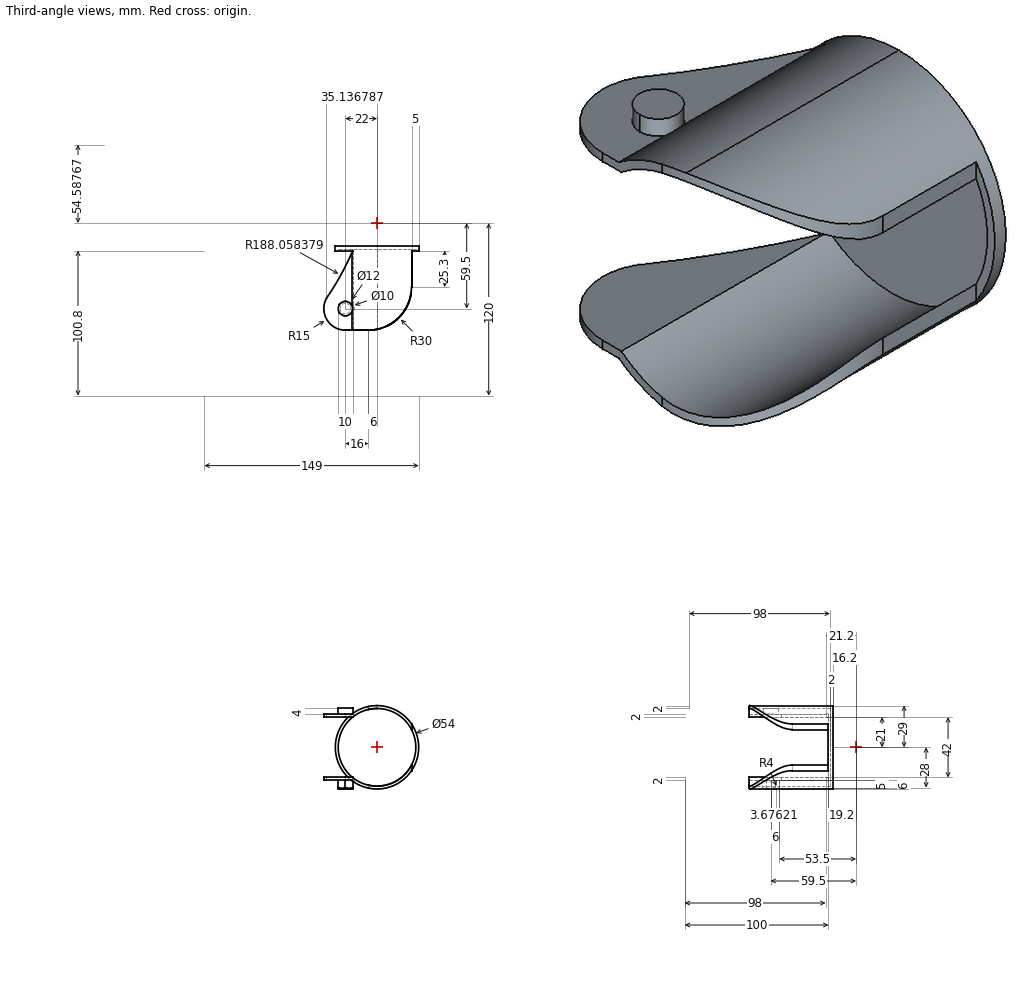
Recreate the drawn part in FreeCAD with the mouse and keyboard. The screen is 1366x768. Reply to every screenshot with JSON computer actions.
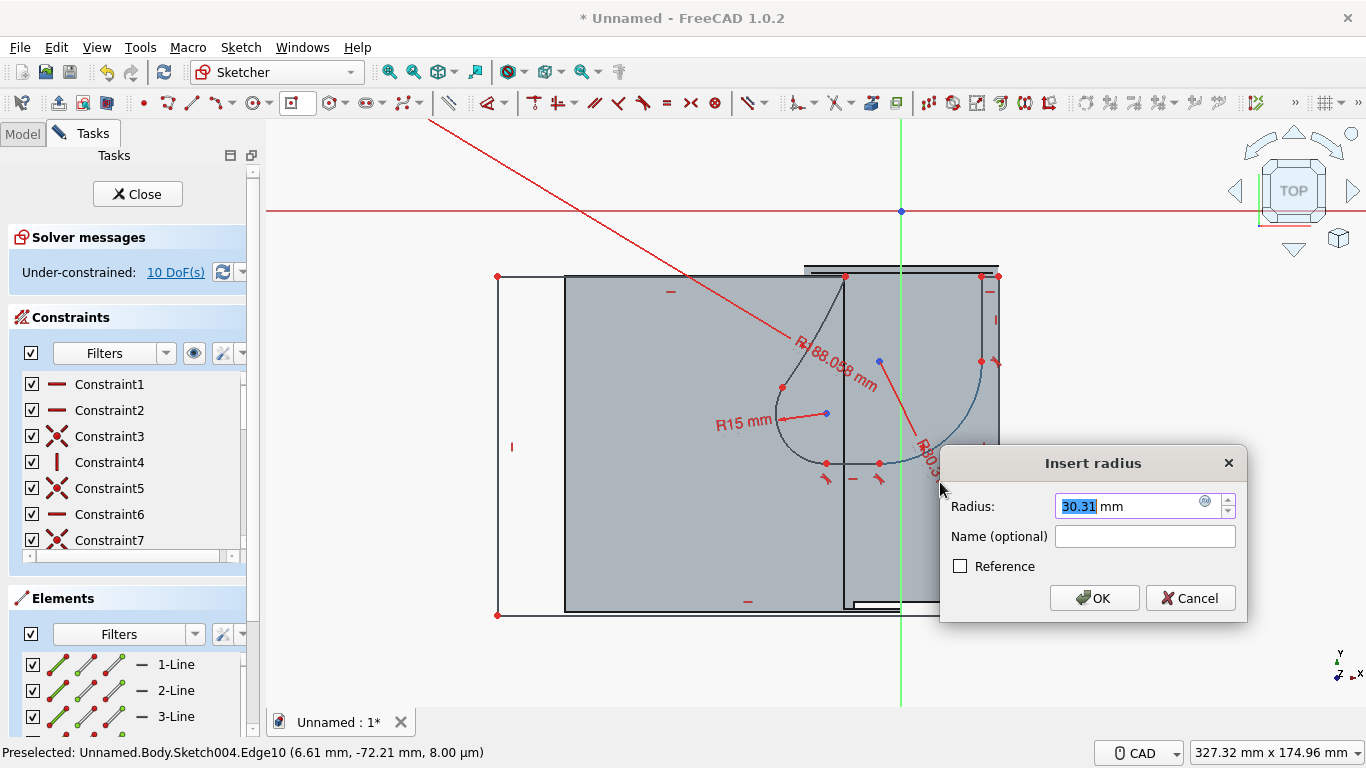
{"action": "type", "text": "30"}
{"action": "key", "text": "Return"}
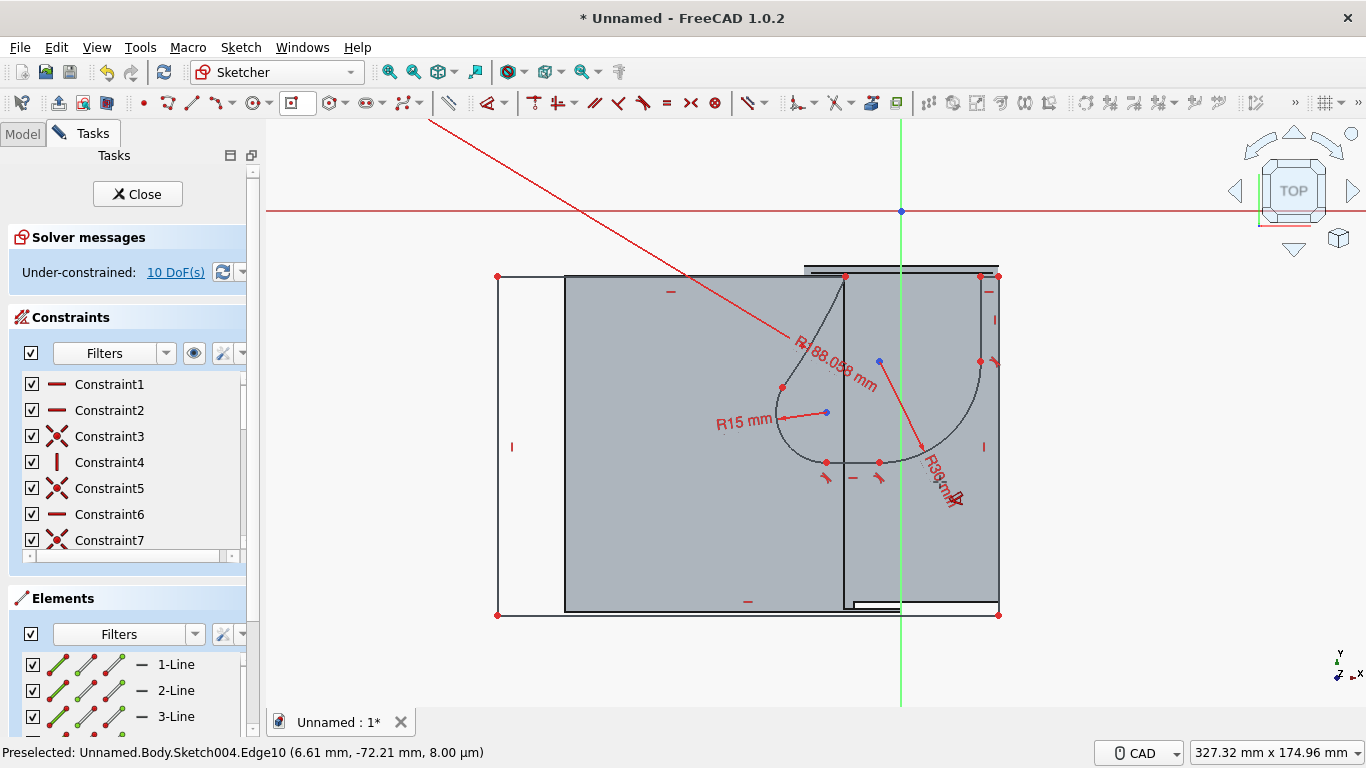
{"action": "scroll", "coordinate": [990, 277], "scroll_direction": "up", "scroll_amount": 5}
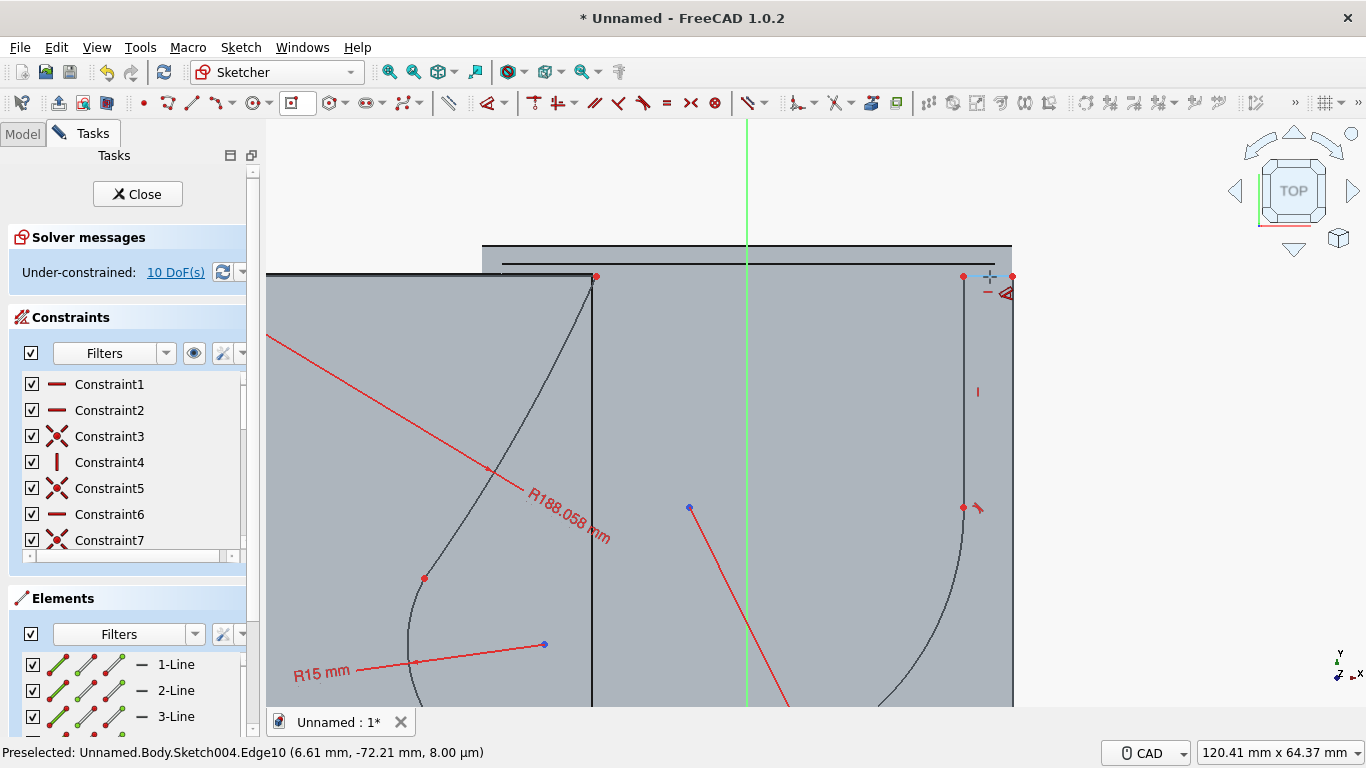
{"action": "left_click", "coordinate": [988, 276]}
{"action": "left_click", "coordinate": [988, 242]}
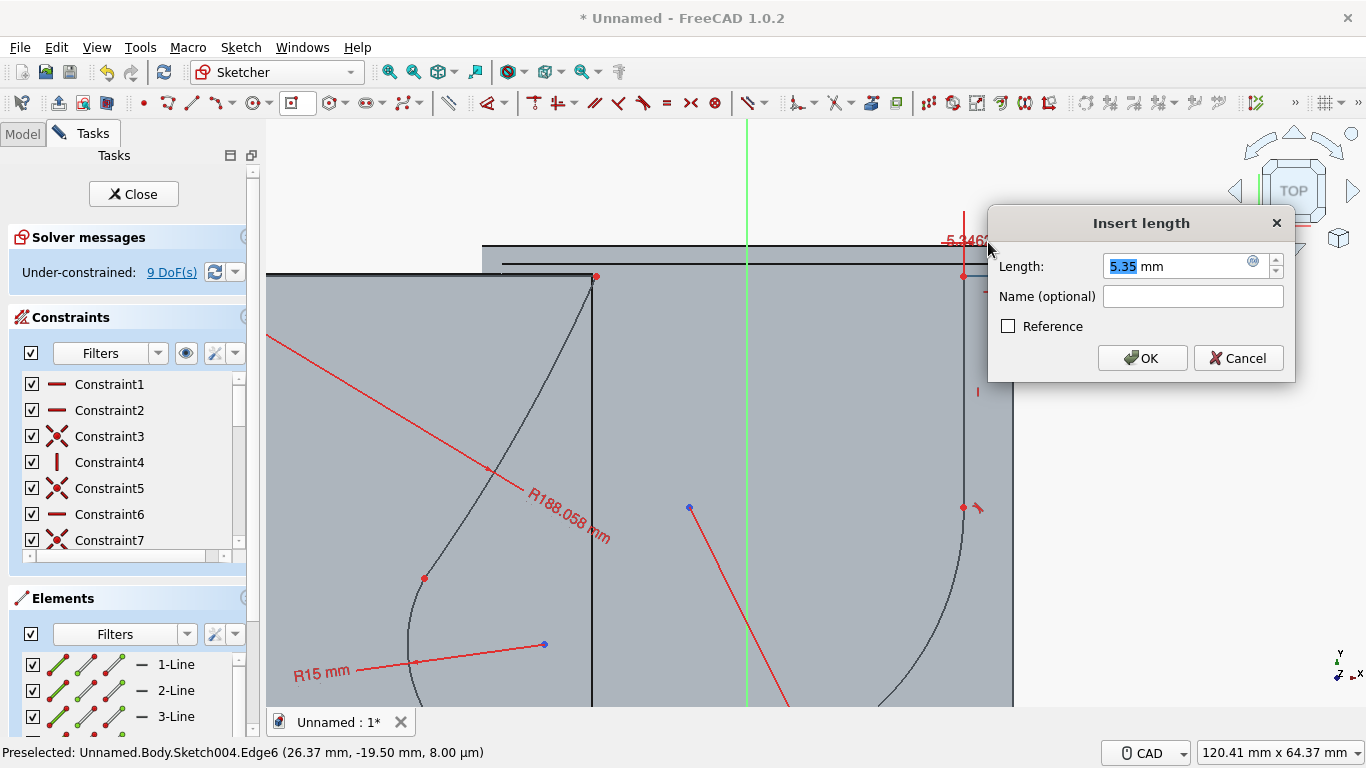
{"action": "type", "text": "5"}
{"action": "key", "text": "Return"}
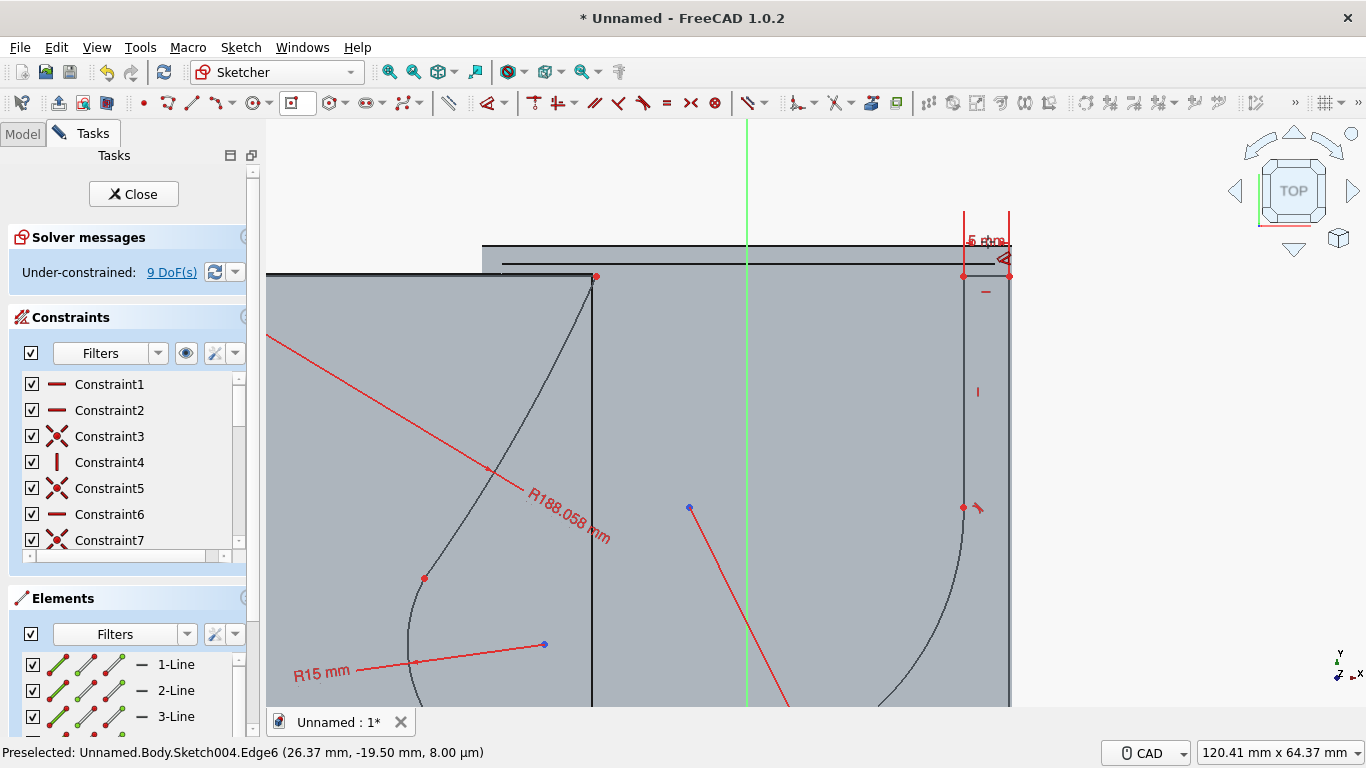
{"action": "scroll", "coordinate": [990, 277], "scroll_direction": "down", "scroll_amount": 5}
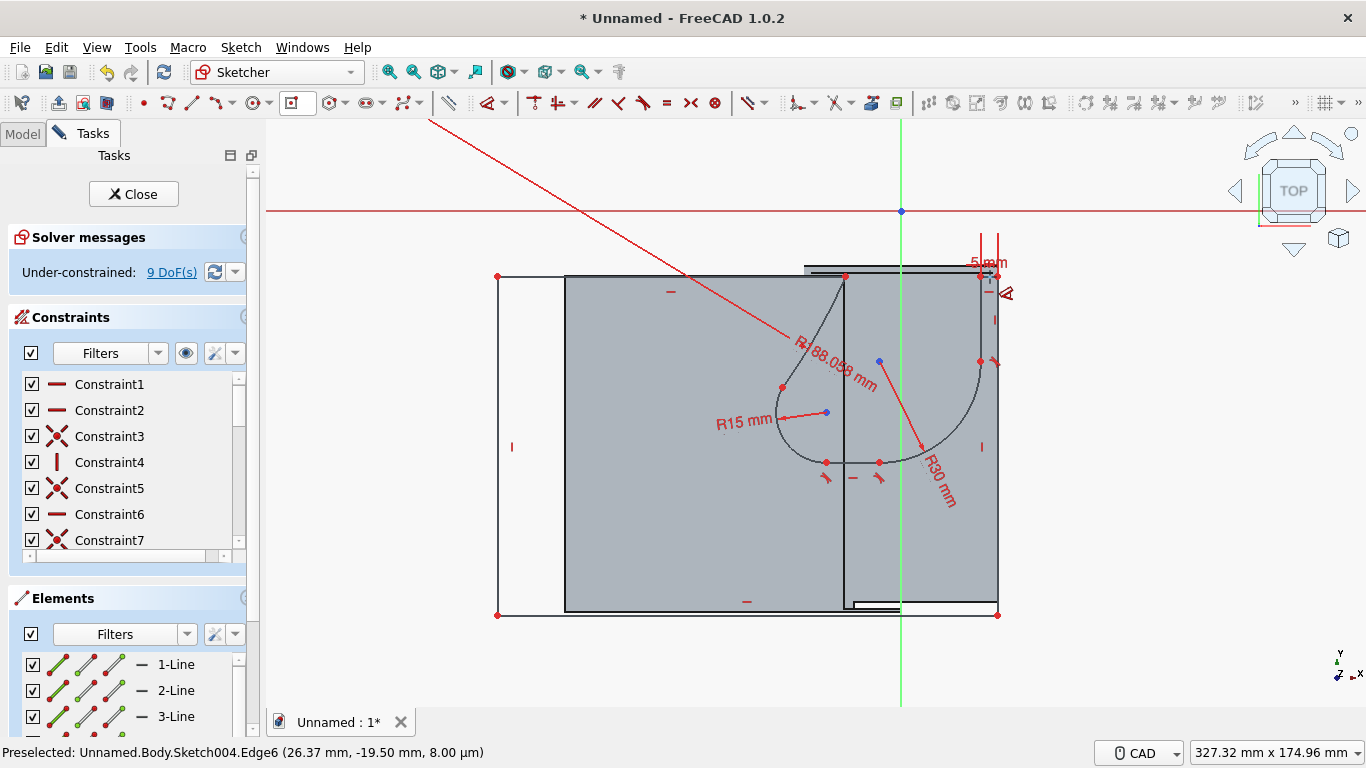
{"action": "left_click", "coordinate": [864, 463]}
{"action": "left_click", "coordinate": [853, 497]}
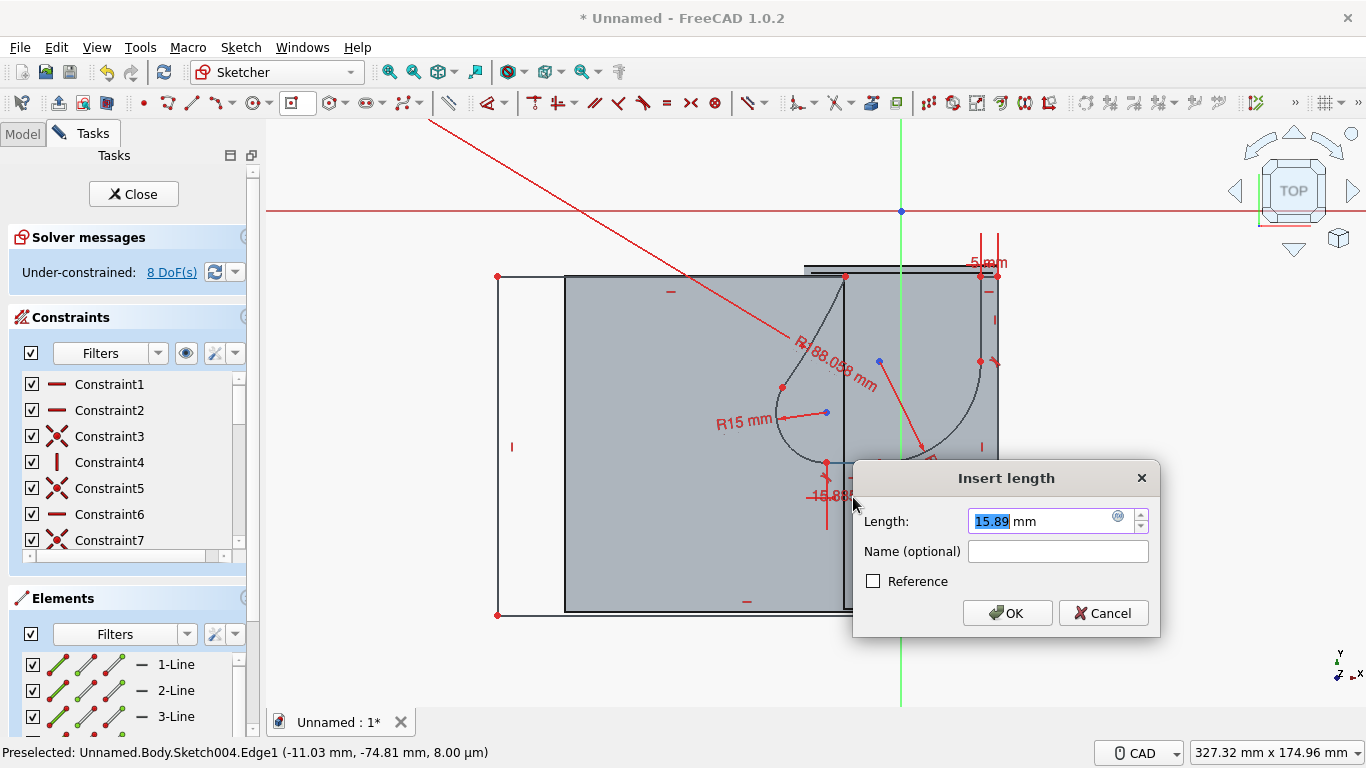
{"action": "type", "text": "16"}
{"action": "key", "text": "Return"}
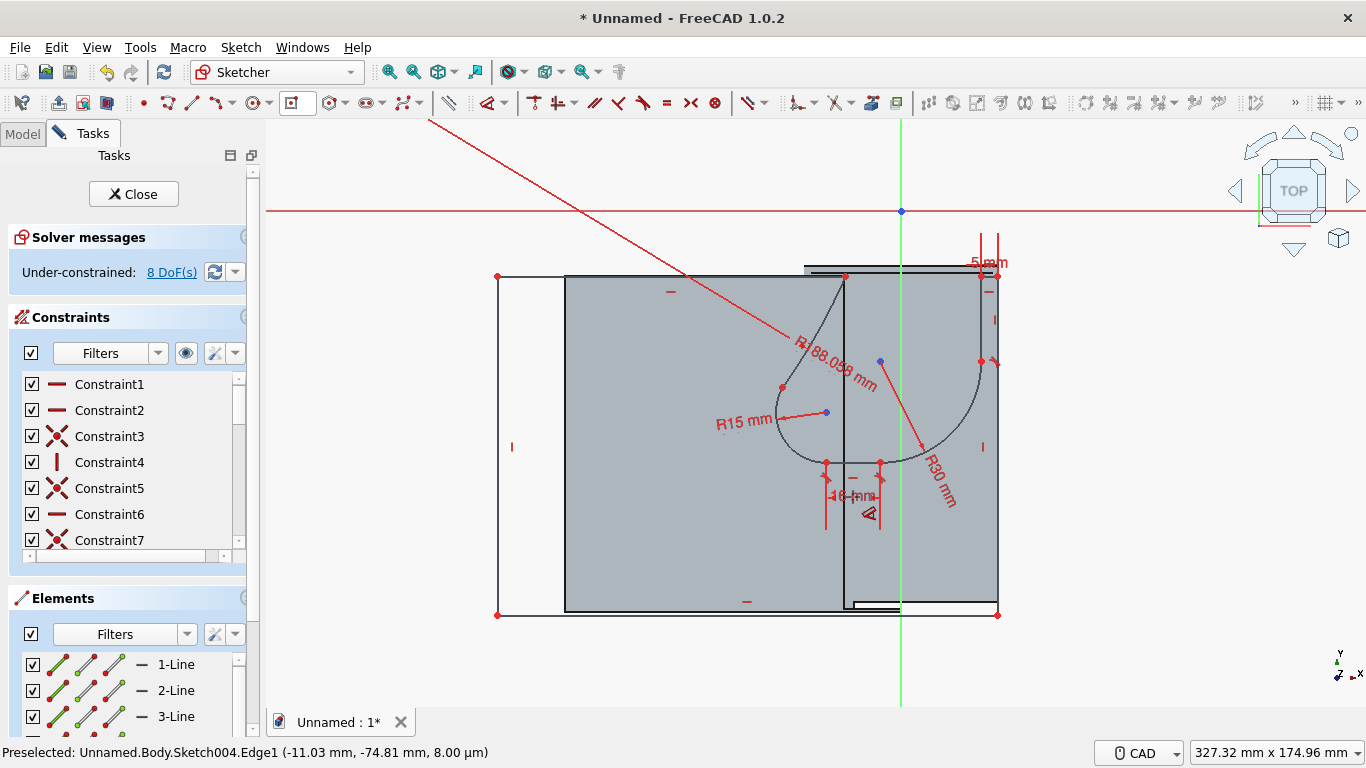
{"action": "scroll", "coordinate": [880, 463], "scroll_direction": "up", "scroll_amount": 4}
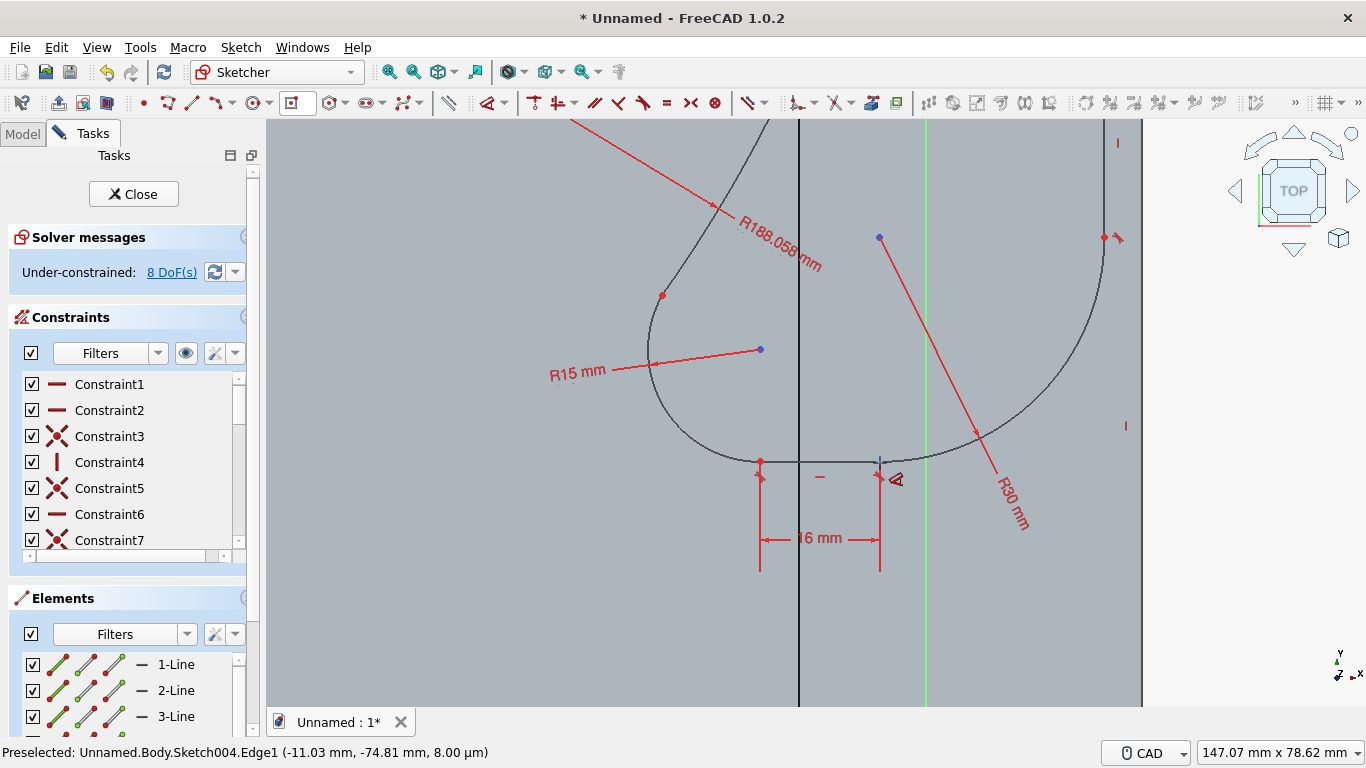
{"action": "left_click", "coordinate": [880, 462]}
{"action": "left_click", "coordinate": [903, 496]}